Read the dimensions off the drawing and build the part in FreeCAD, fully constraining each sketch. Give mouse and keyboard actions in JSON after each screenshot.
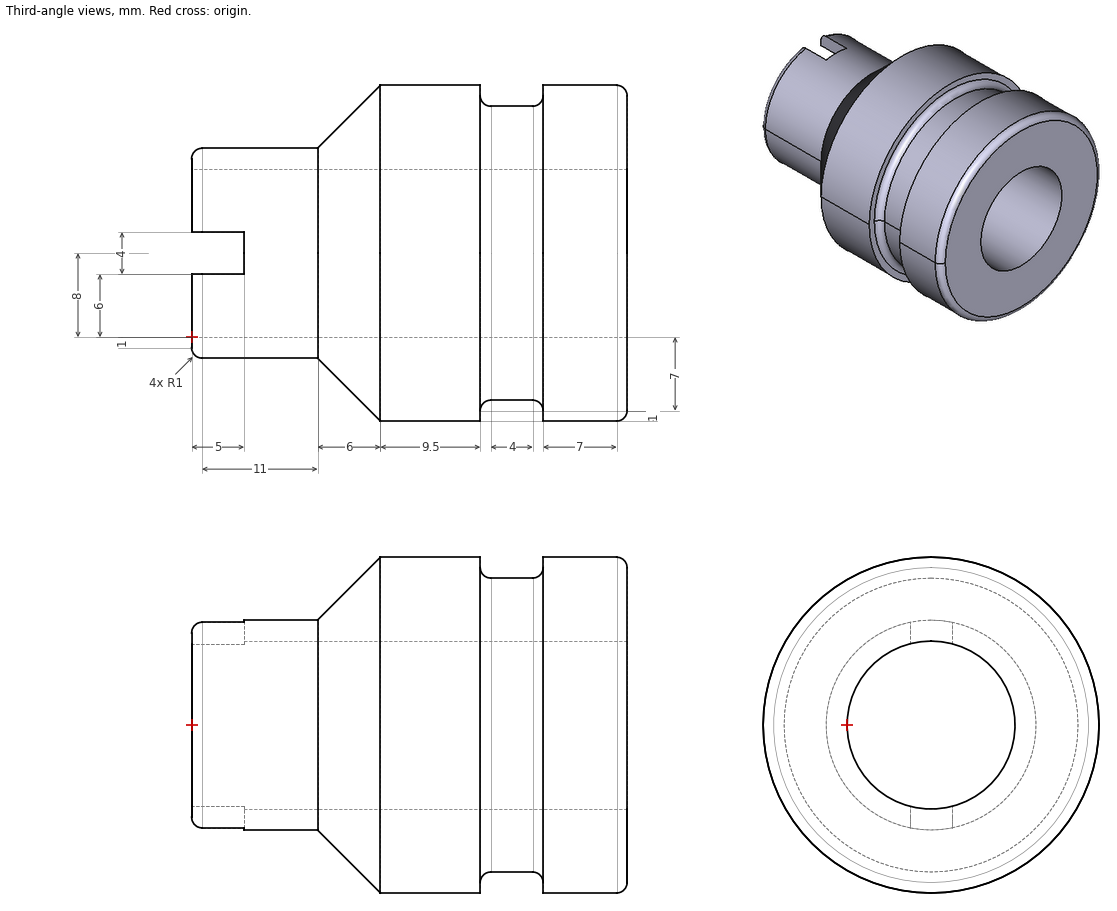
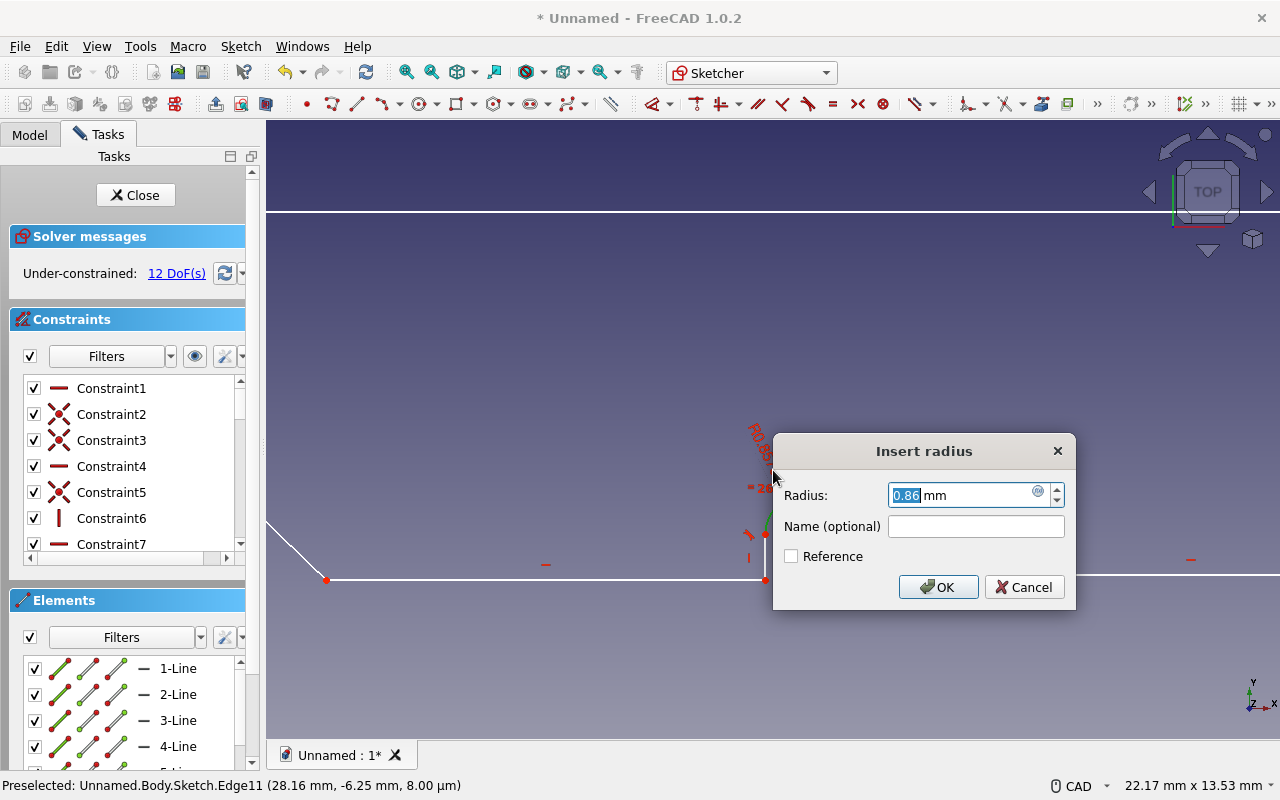
{"action": "type", "text": "1"}
{"action": "key", "text": "Return"}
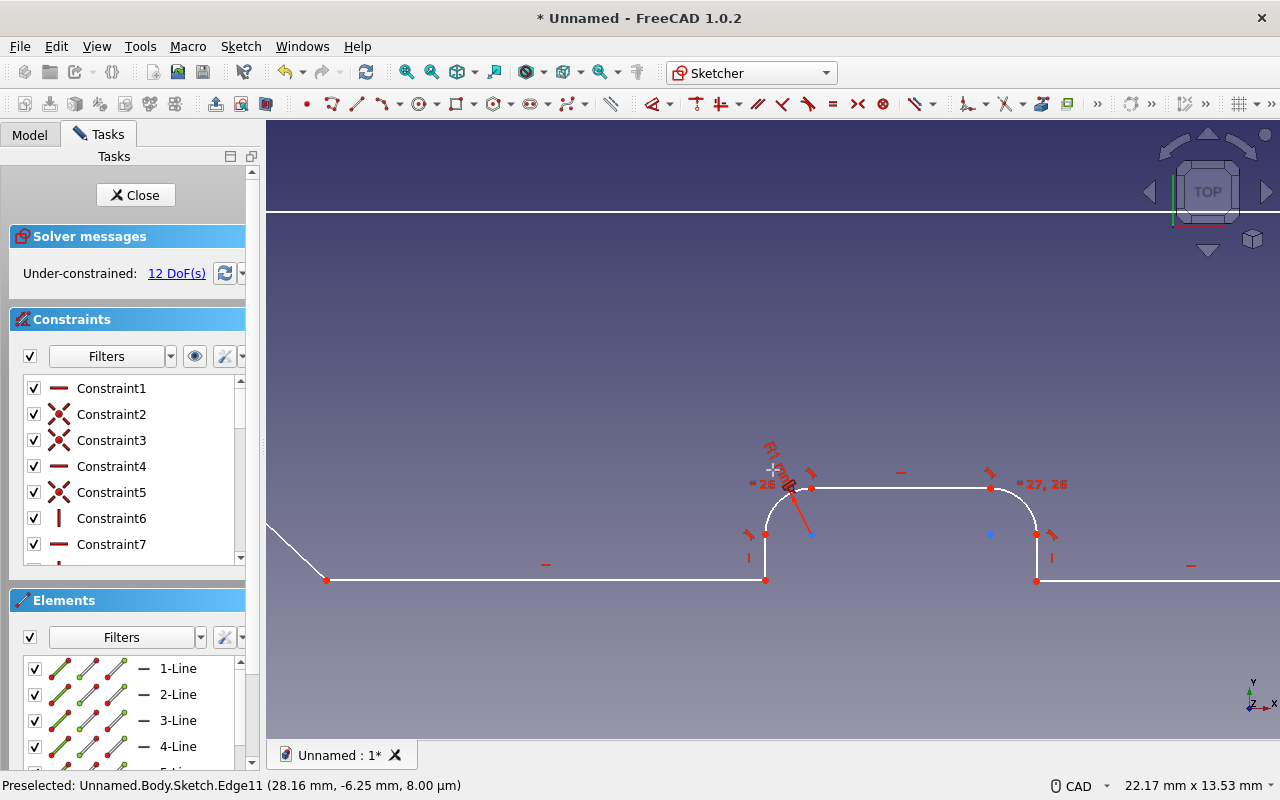
{"action": "left_click", "coordinate": [765, 567]}
{"action": "left_click", "coordinate": [799, 557]}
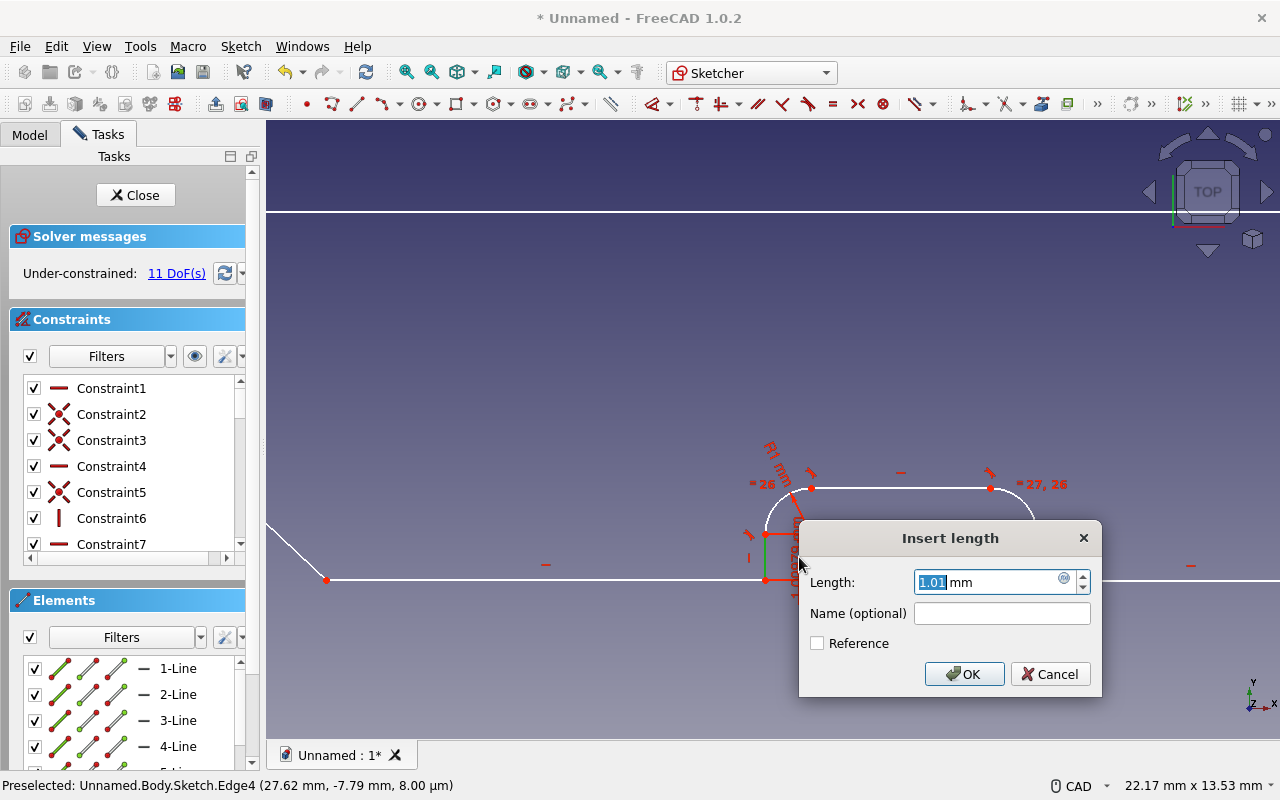
{"action": "type", "text": "1"}
{"action": "key", "text": "Return"}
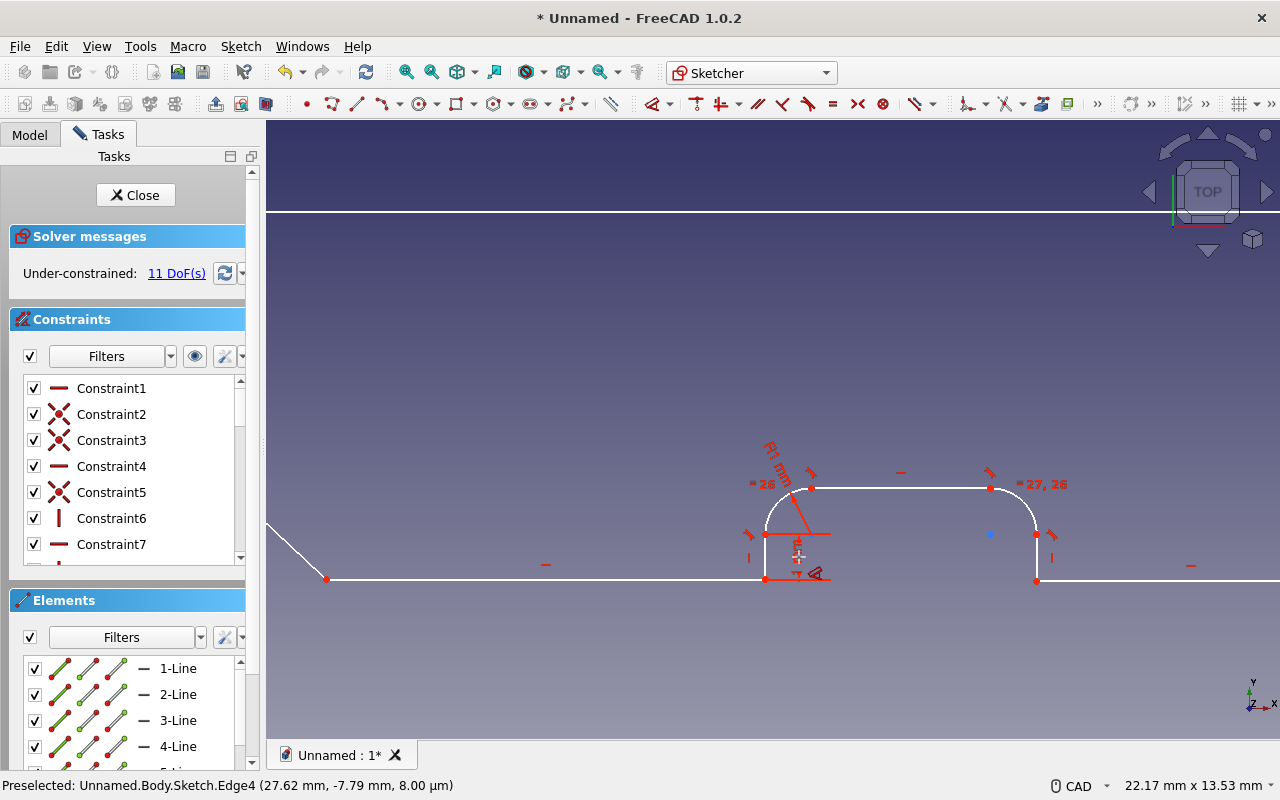
{"action": "scroll", "coordinate": [787, 501], "scroll_direction": "down", "scroll_amount": 7}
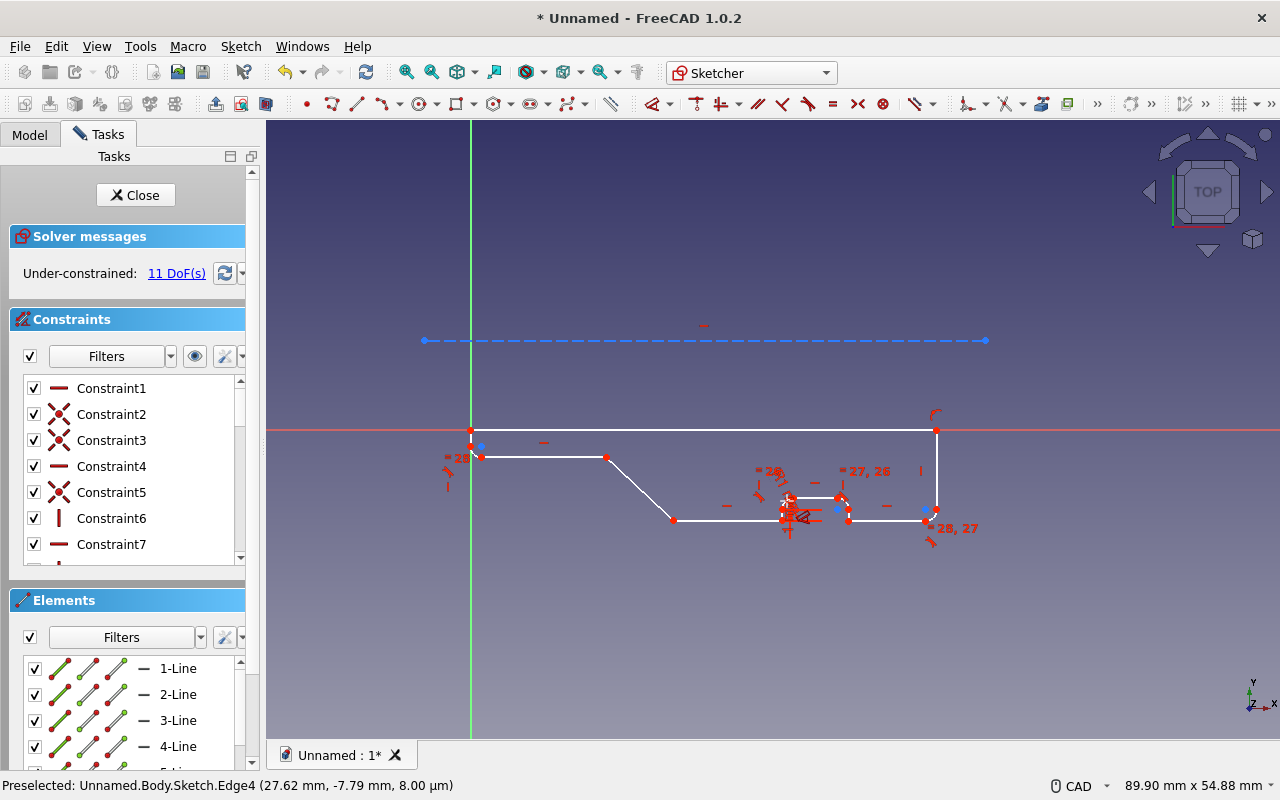
{"action": "left_click", "coordinate": [807, 498]}
{"action": "left_click", "coordinate": [816, 464]}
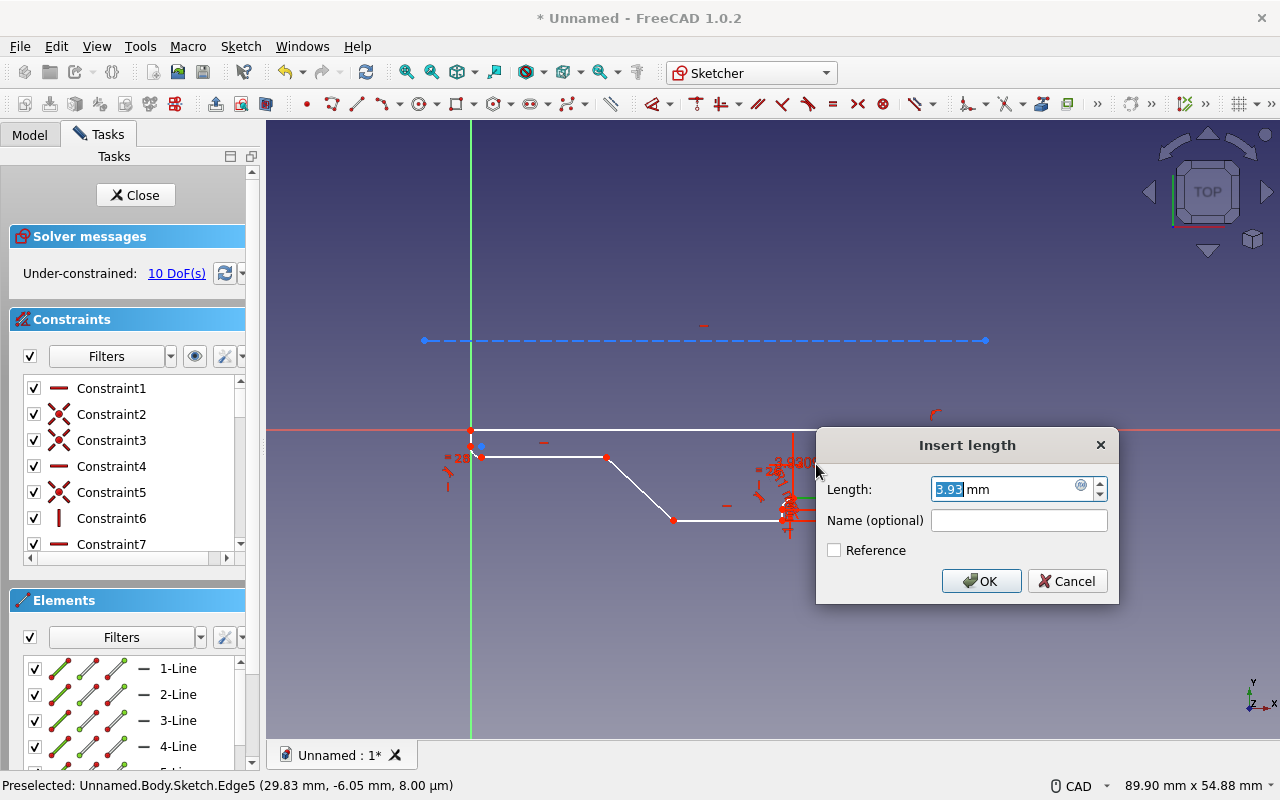
{"action": "type", "text": "4"}
{"action": "key", "text": "Return"}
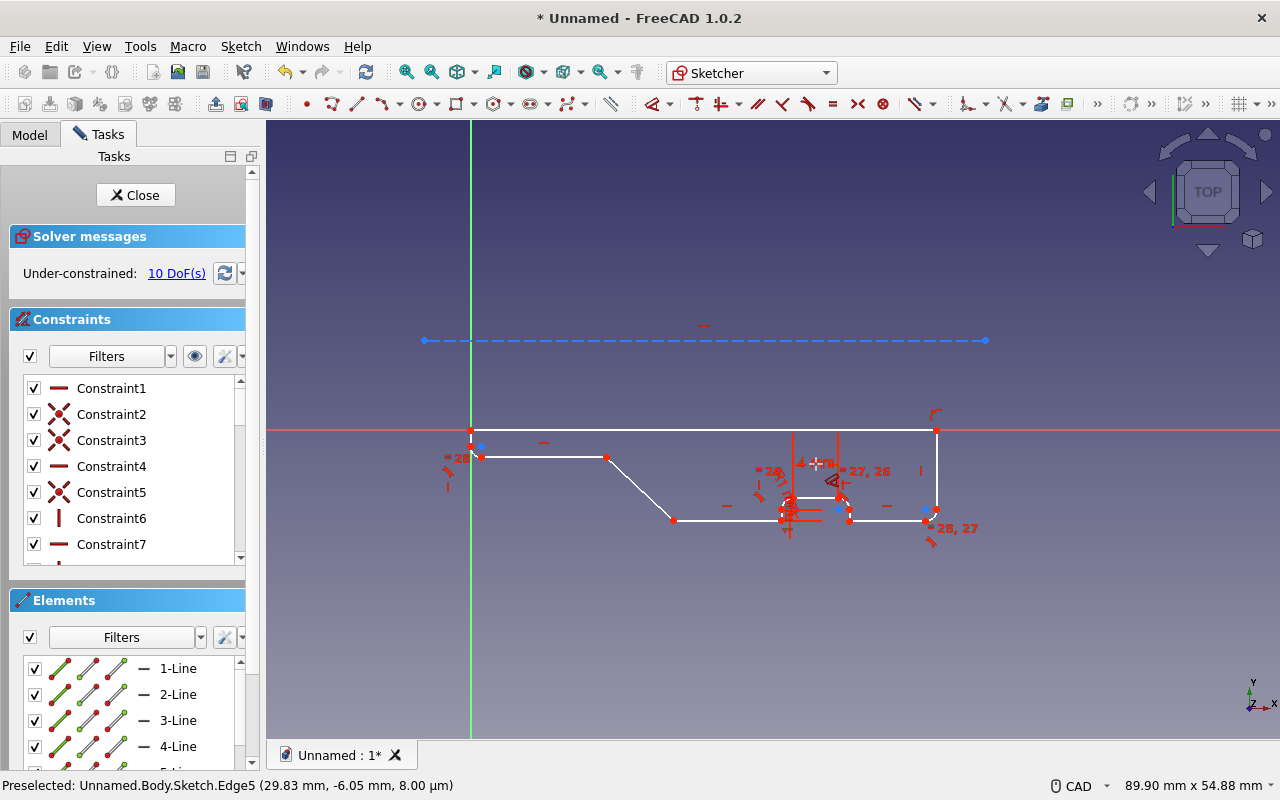
{"action": "scroll", "coordinate": [850, 515], "scroll_direction": "up", "scroll_amount": 7}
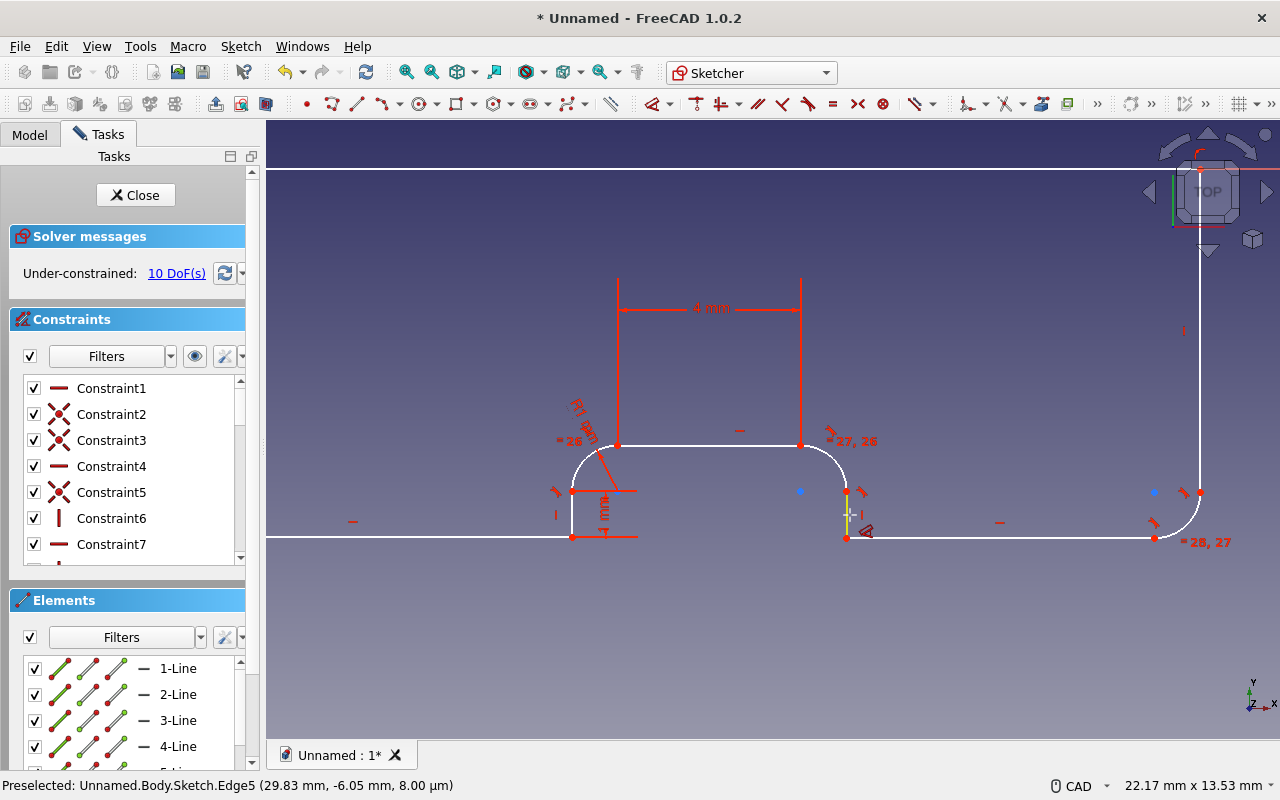
{"action": "left_click", "coordinate": [847, 515]}
{"action": "left_click", "coordinate": [881, 515]}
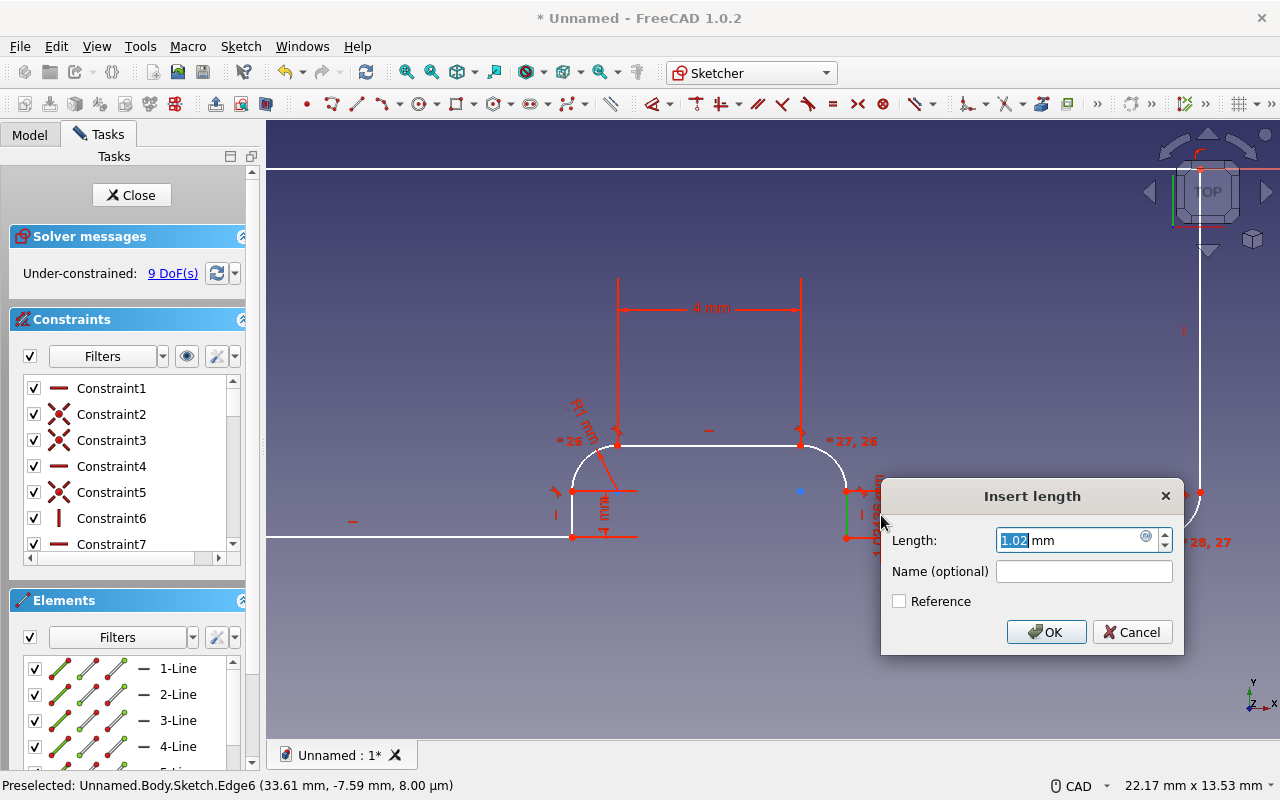
{"action": "type", "text": "1"}
{"action": "key", "text": "Return"}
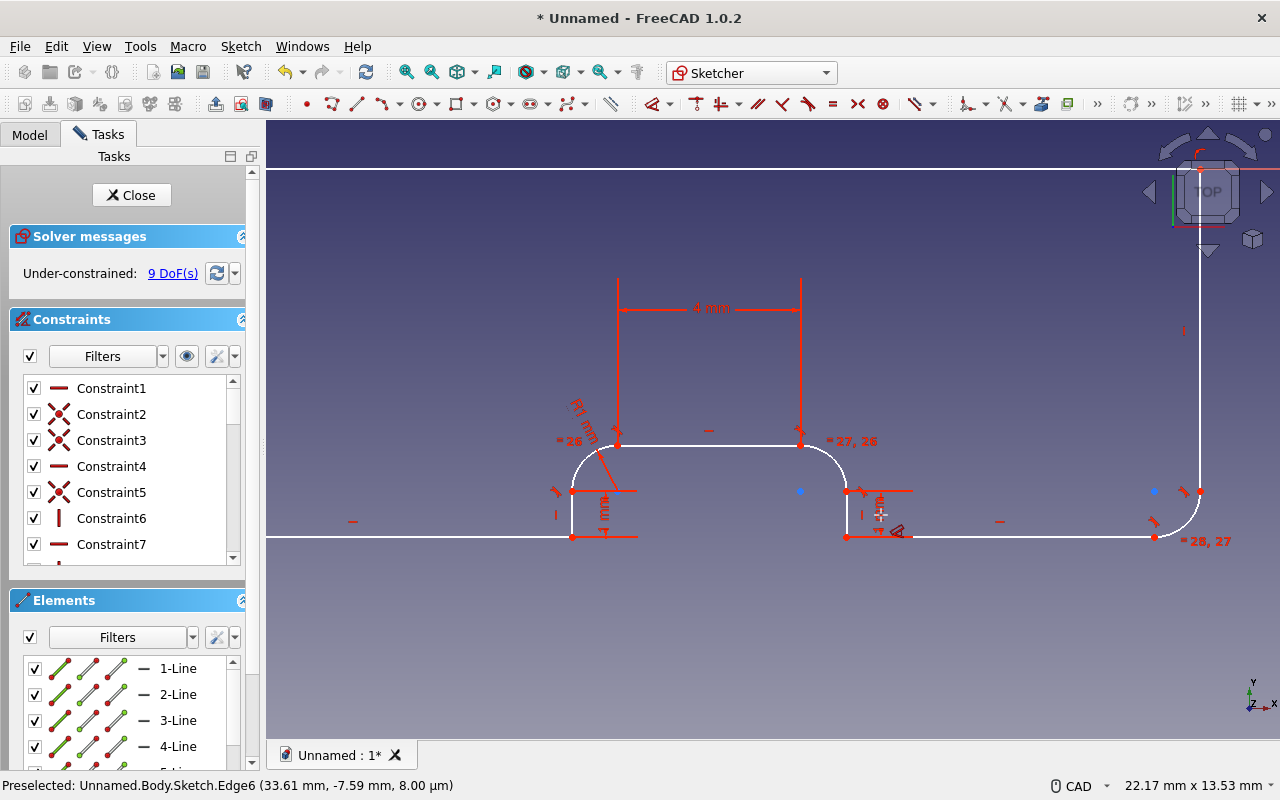
{"action": "scroll", "coordinate": [850, 515], "scroll_direction": "down", "scroll_amount": 7}